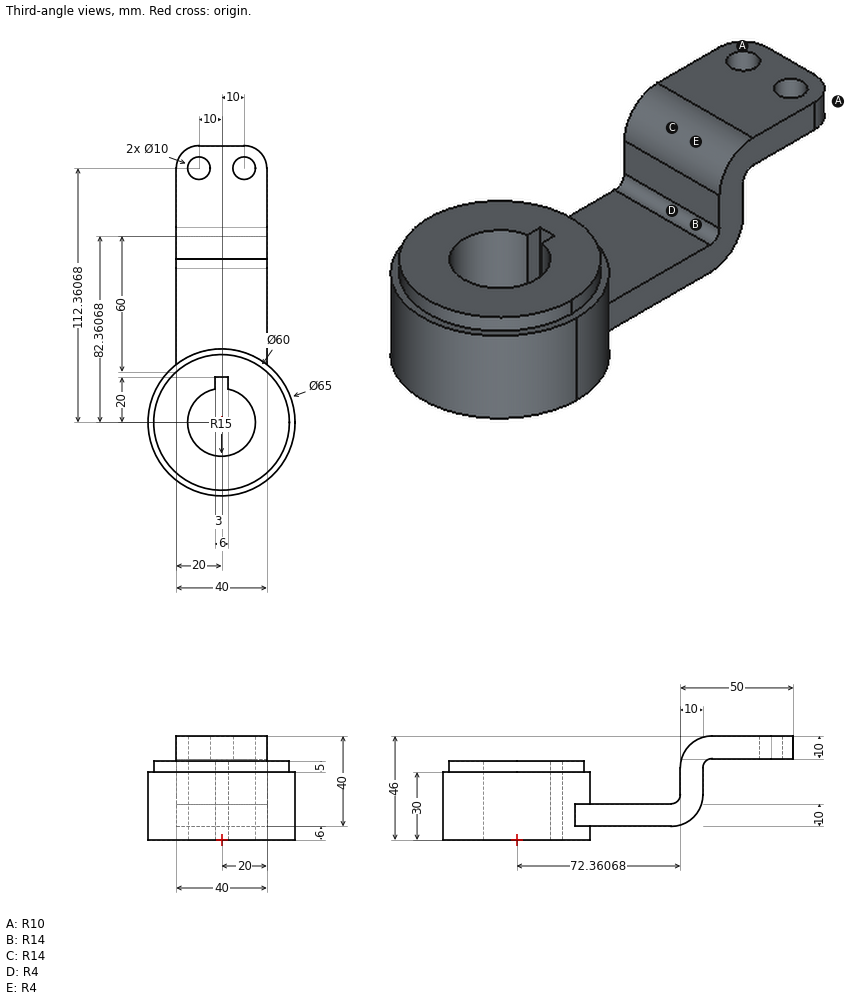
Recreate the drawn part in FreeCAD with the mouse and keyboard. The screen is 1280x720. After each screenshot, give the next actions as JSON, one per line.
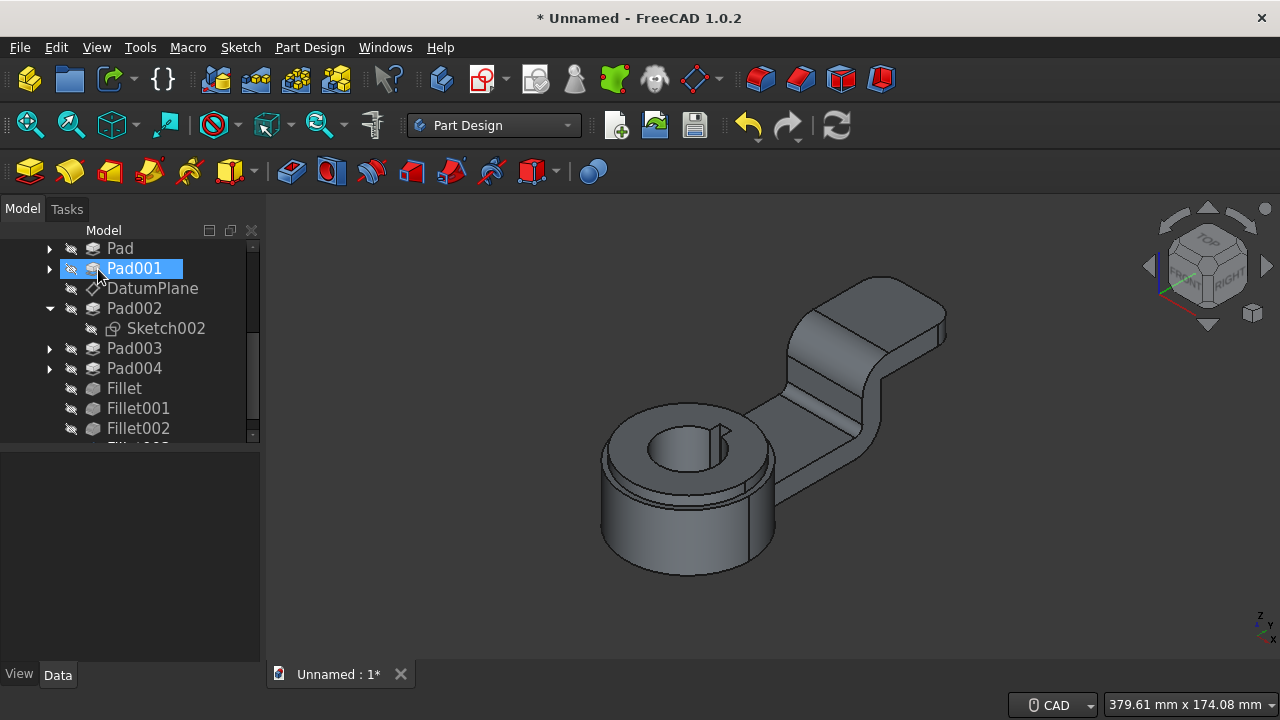
{"action": "key", "text": "1"}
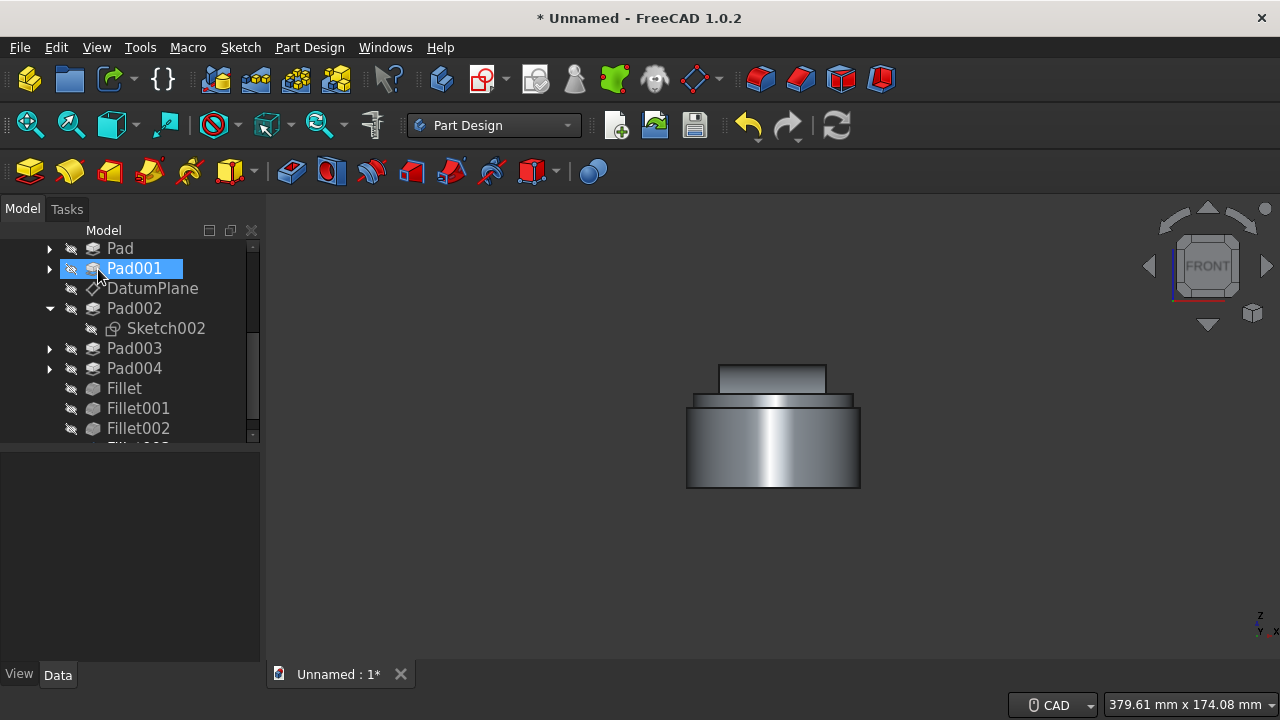
{"action": "key", "text": "v f"}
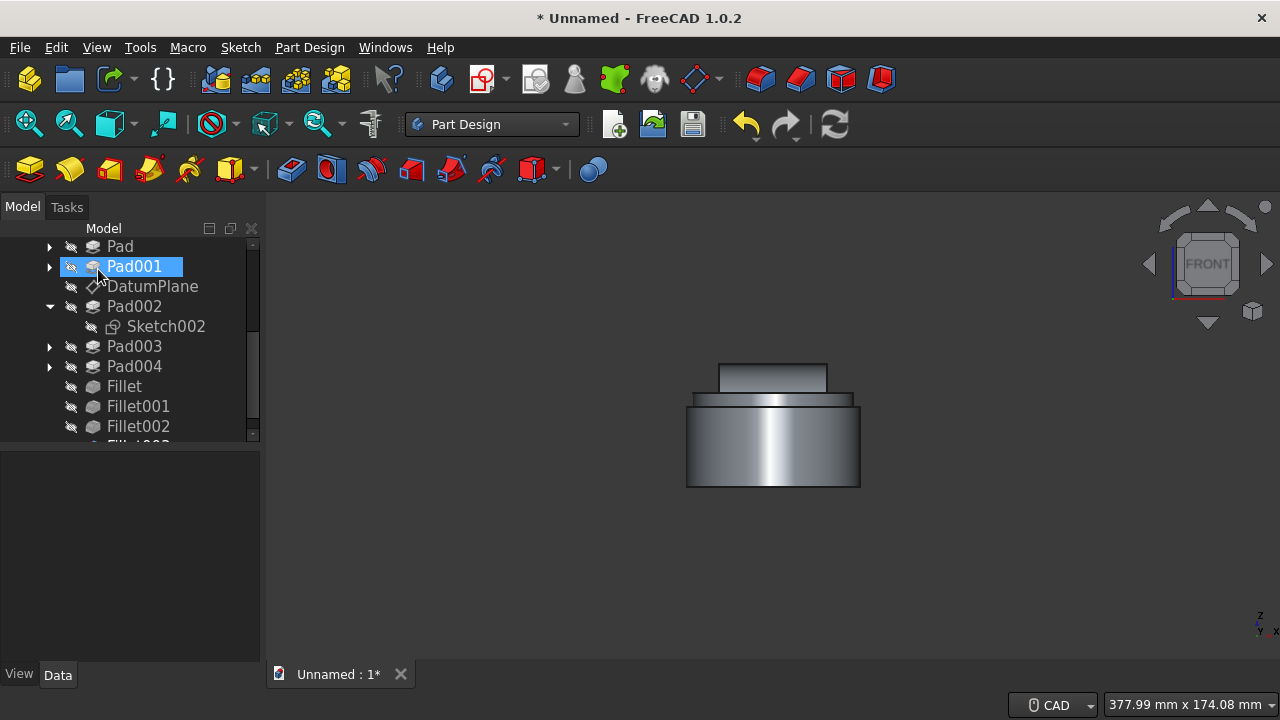
{"action": "key", "text": "3"}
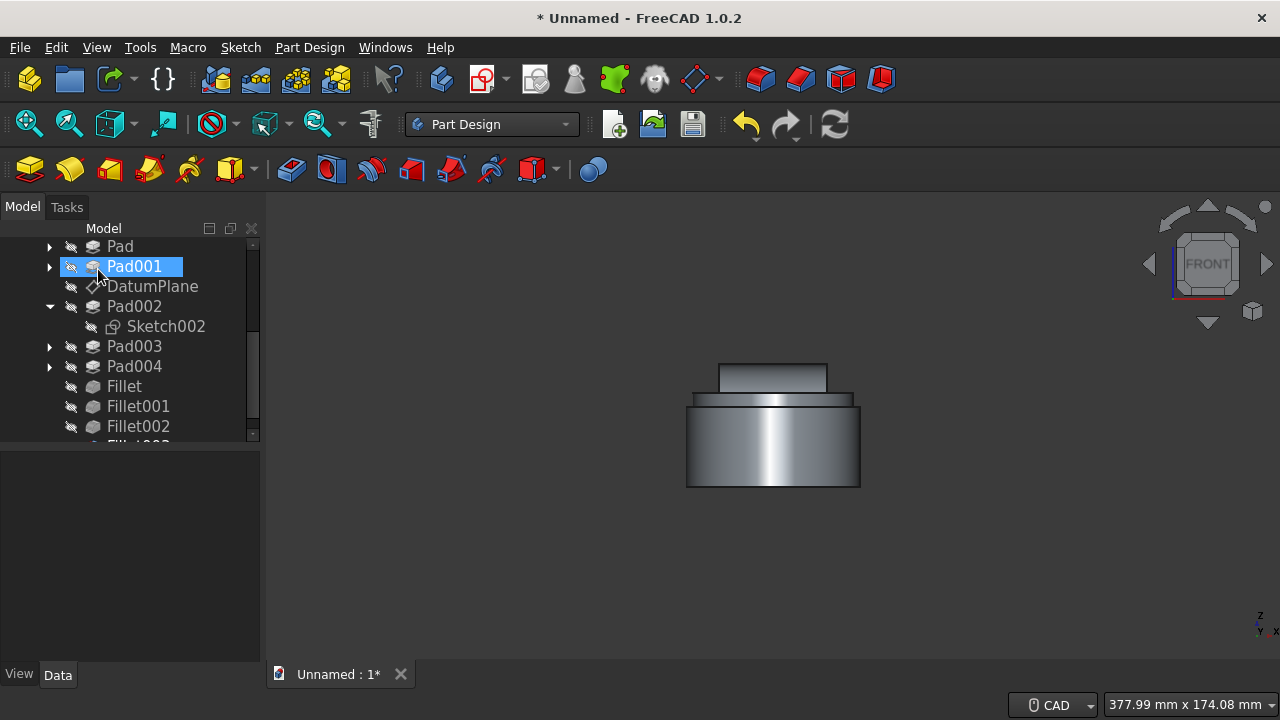
{"action": "left_click", "coordinate": [30, 124]}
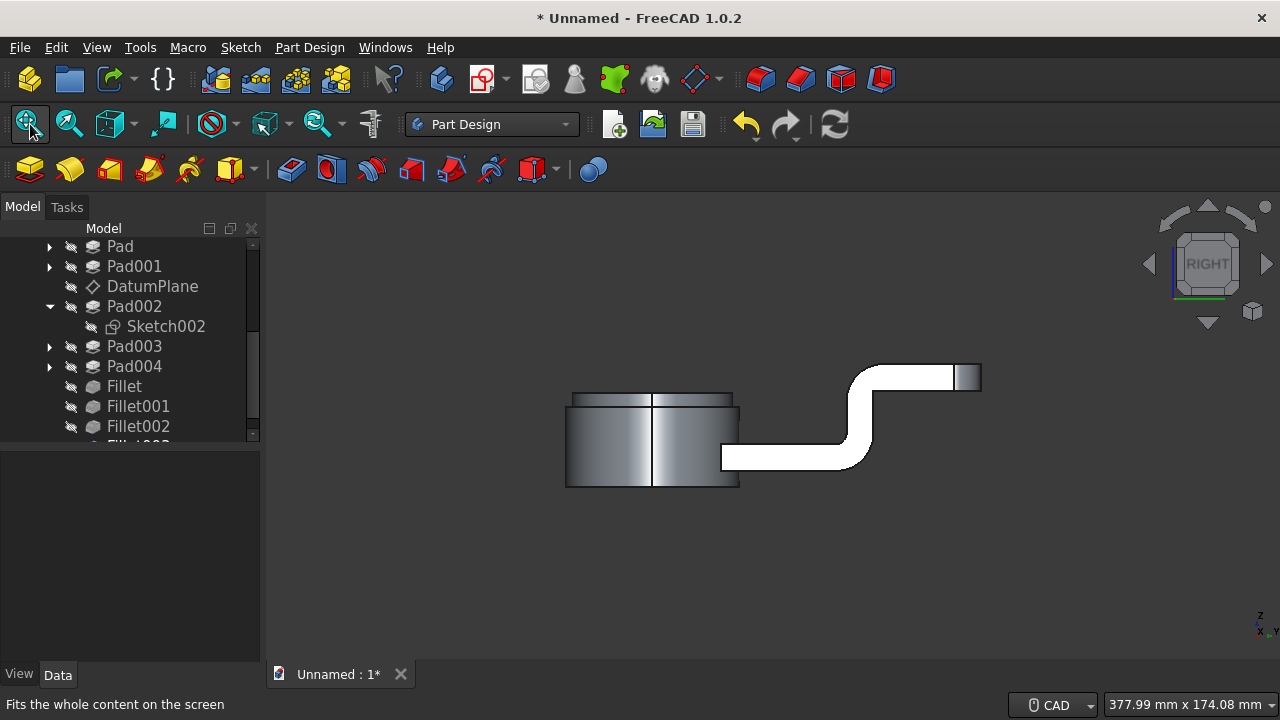
{"action": "key", "text": "5"}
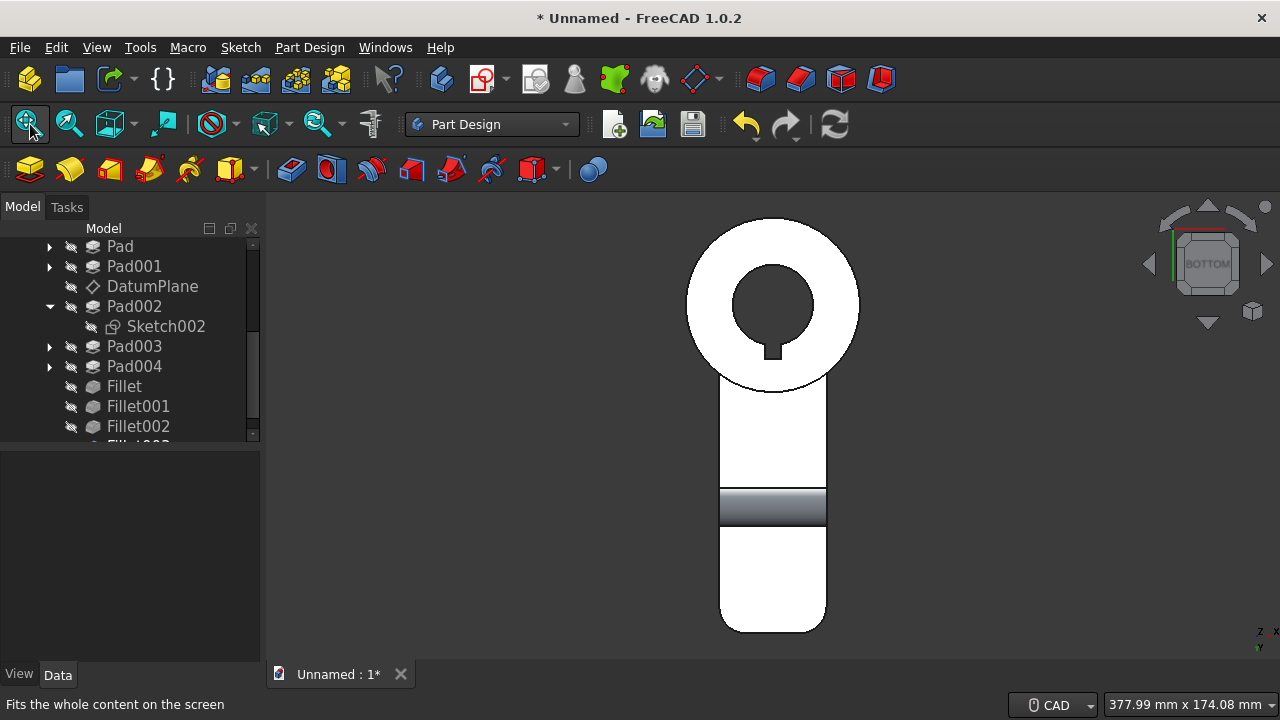
{"action": "key", "text": "4"}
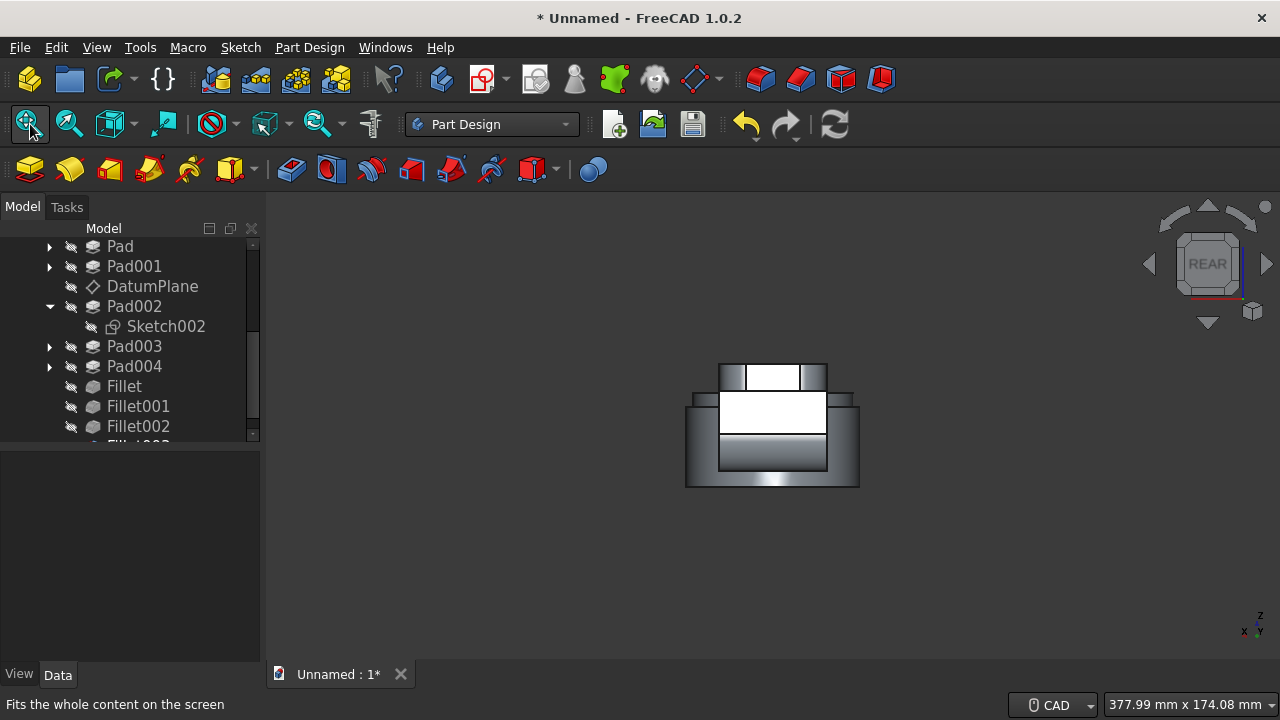
{"action": "key", "text": "v f"}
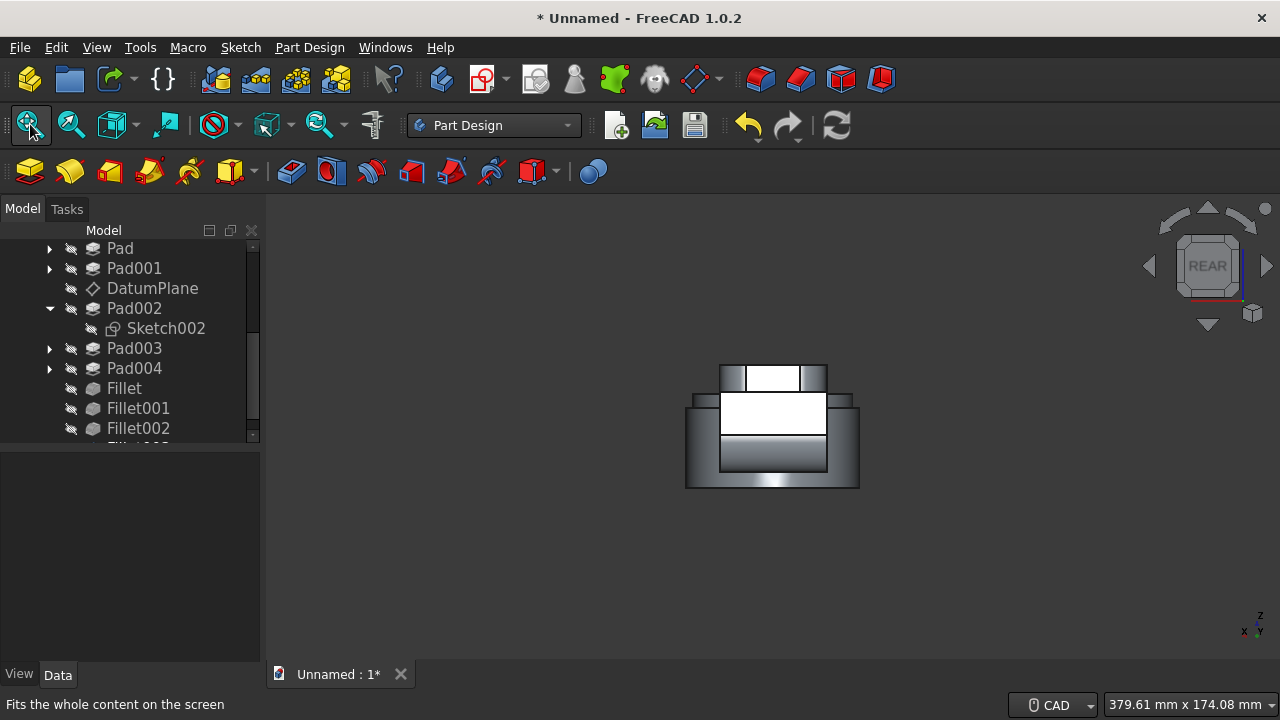
{"action": "key", "text": "6"}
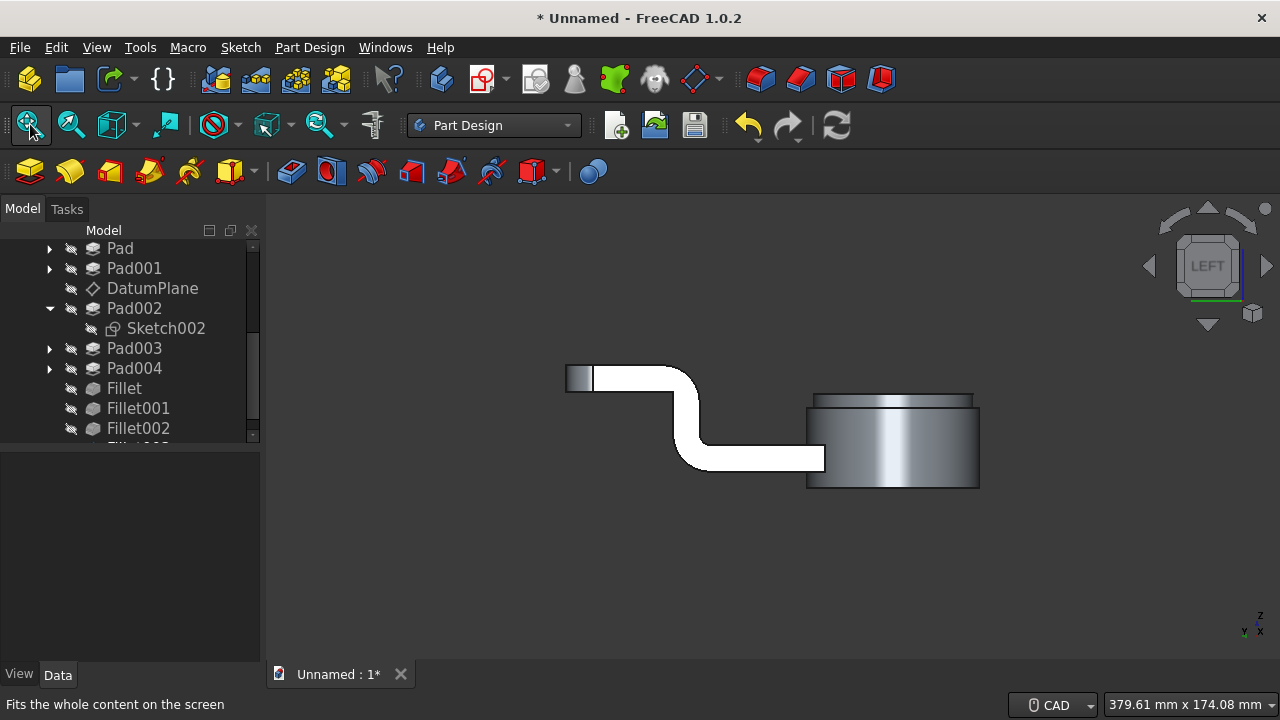
{"action": "key", "text": "v f"}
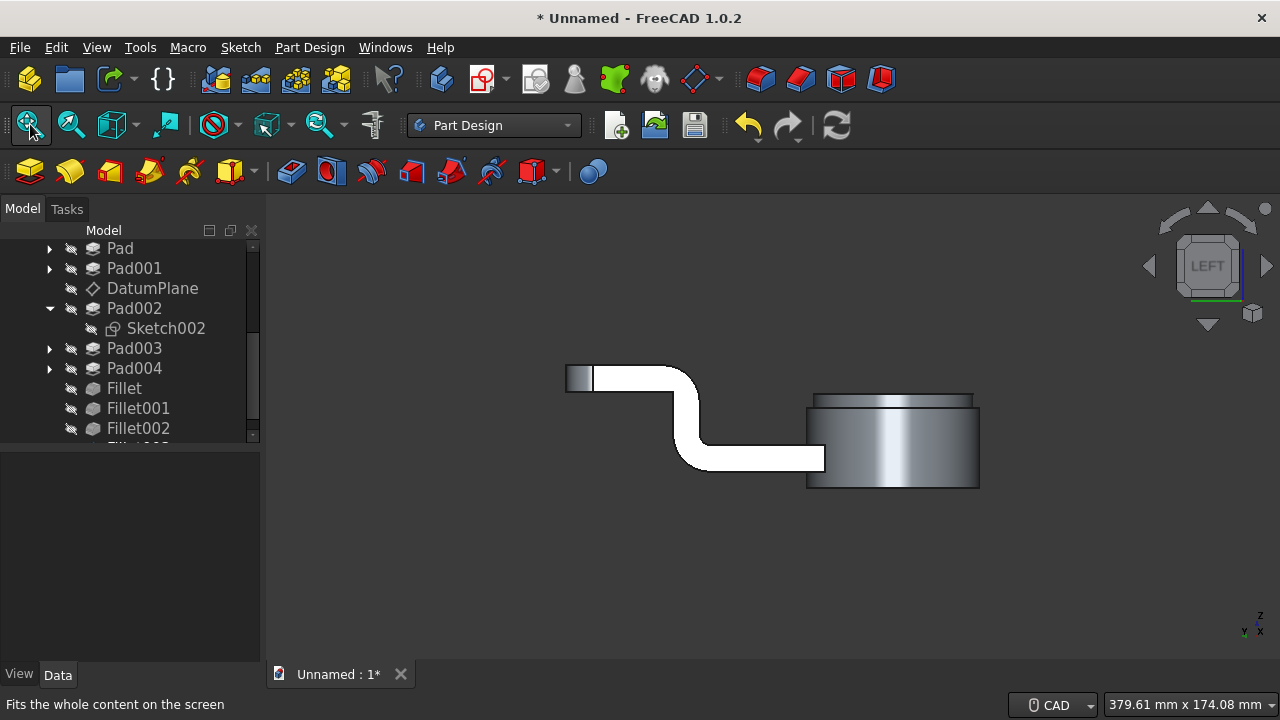
{"action": "key", "text": "v 3"}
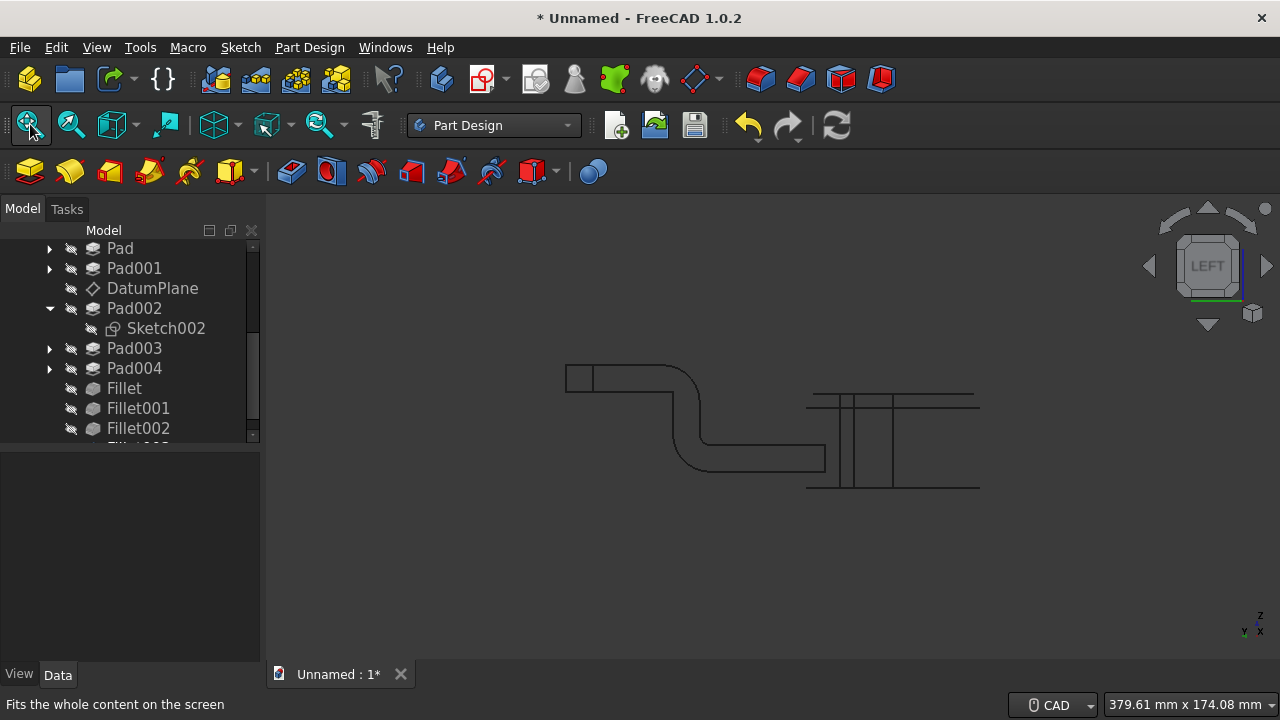
{"action": "key", "text": "0"}